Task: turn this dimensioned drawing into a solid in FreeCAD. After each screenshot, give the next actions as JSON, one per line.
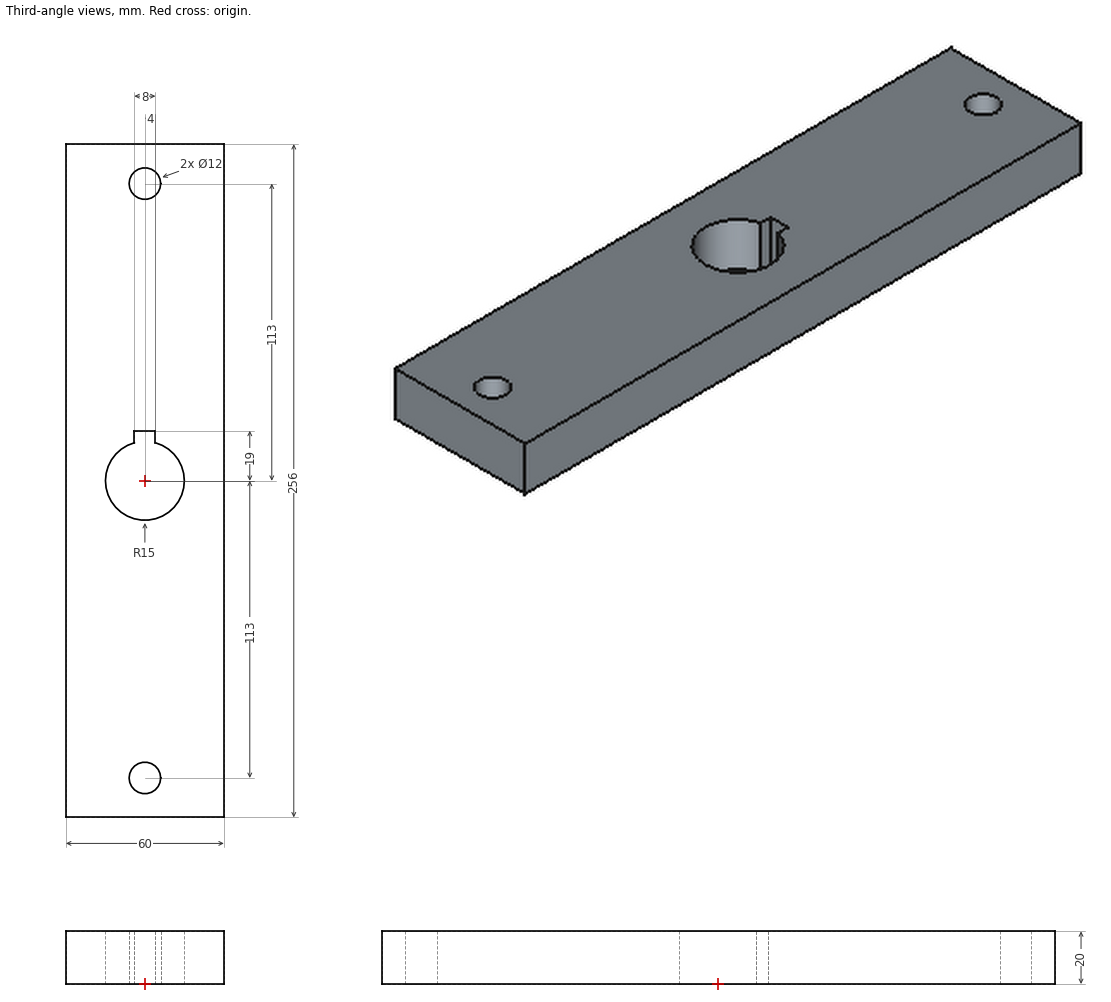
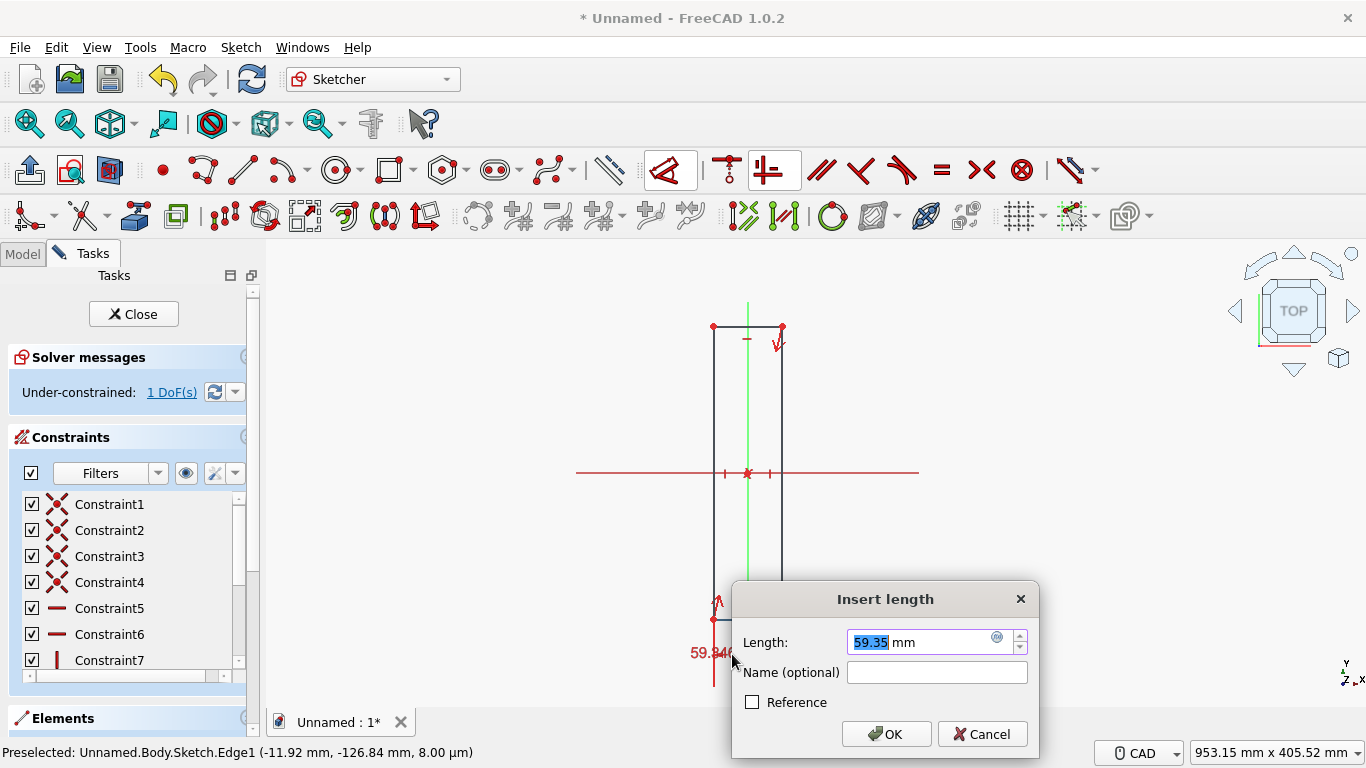
{"action": "type", "text": "60"}
{"action": "key", "text": "Return"}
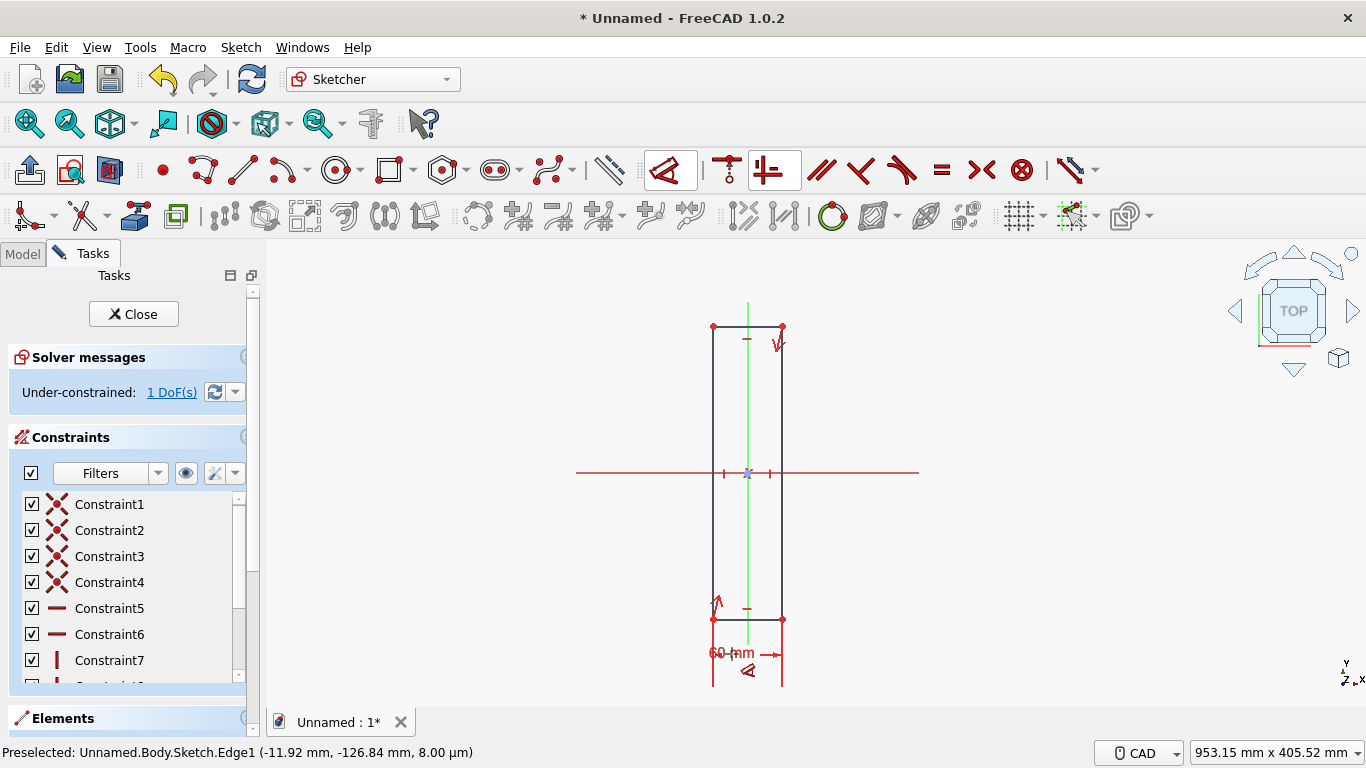
{"action": "left_click", "coordinate": [782, 532]}
{"action": "left_click", "coordinate": [816, 406]}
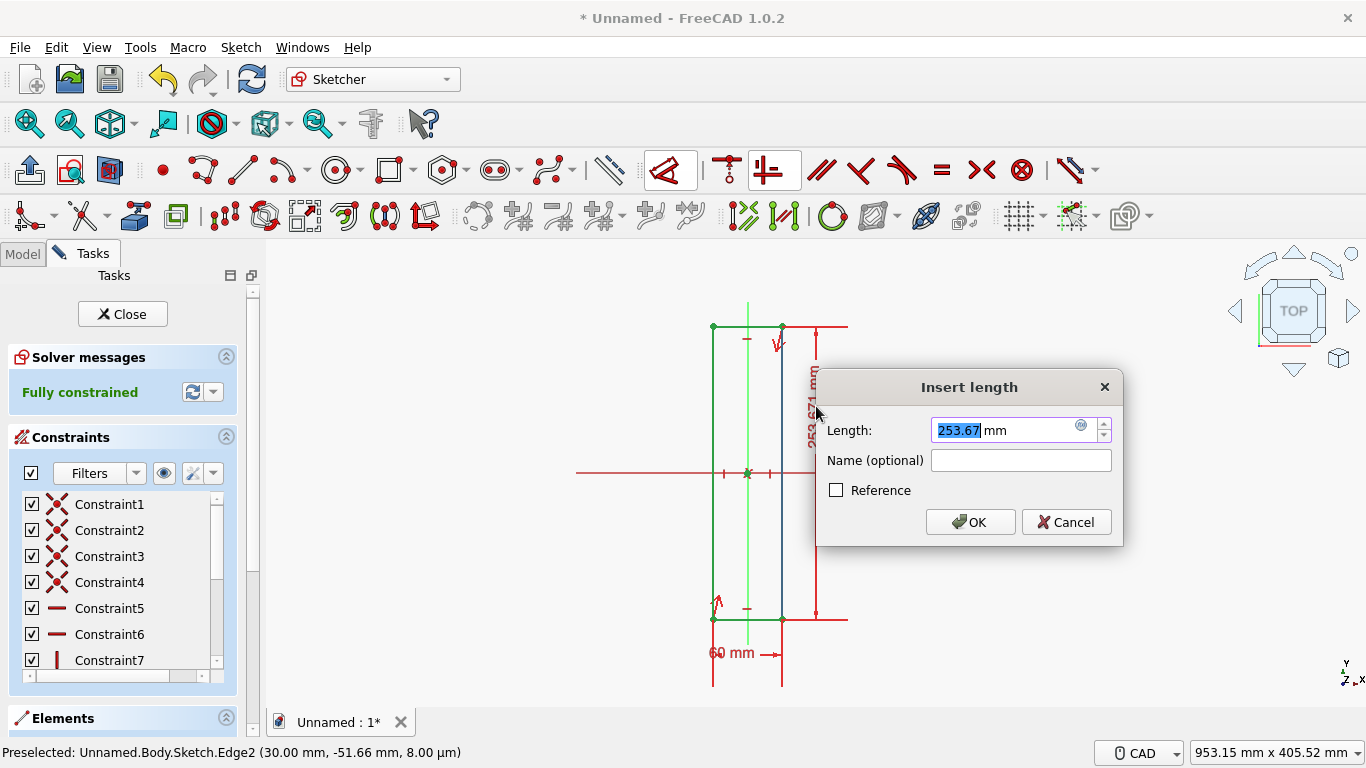
{"action": "type", "text": "256"}
{"action": "key", "text": "Return"}
{"action": "key", "text": "Escape"}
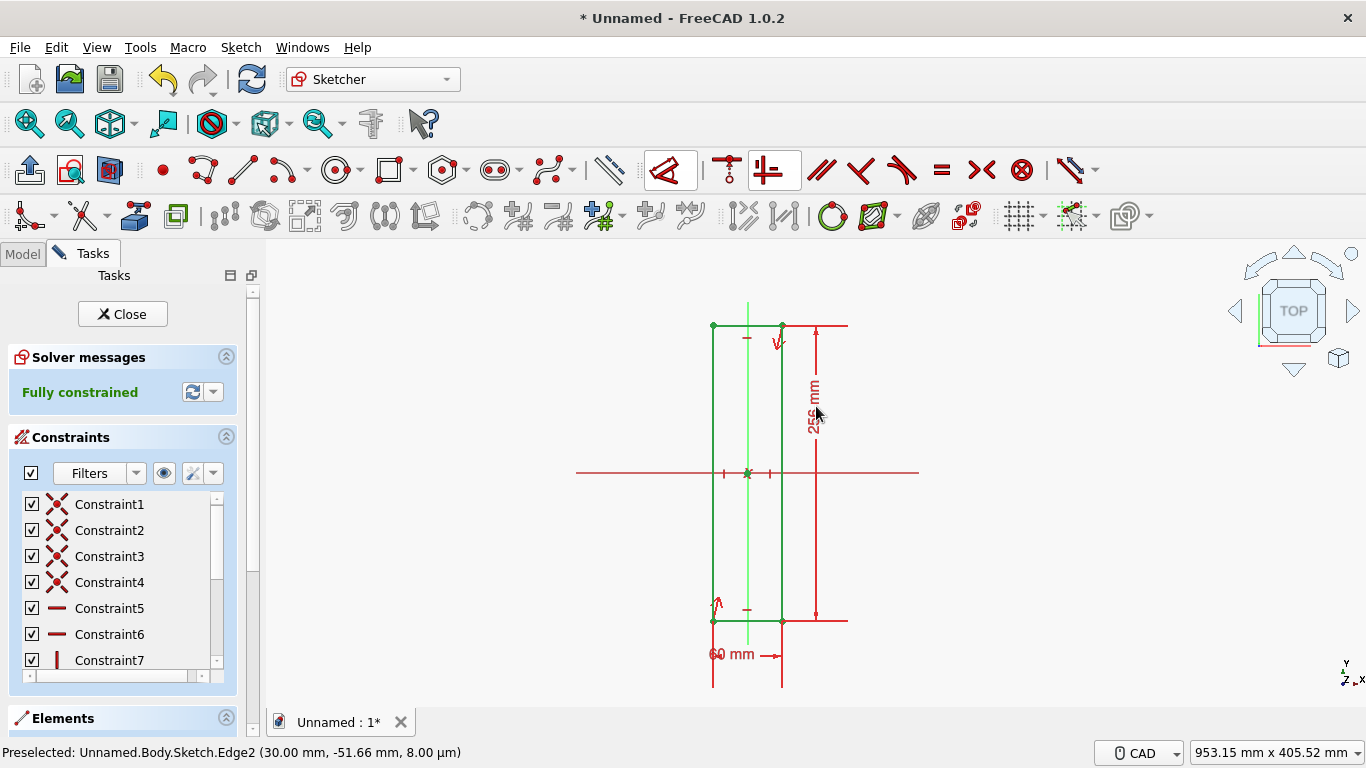
{"action": "left_click", "coordinate": [123, 314]}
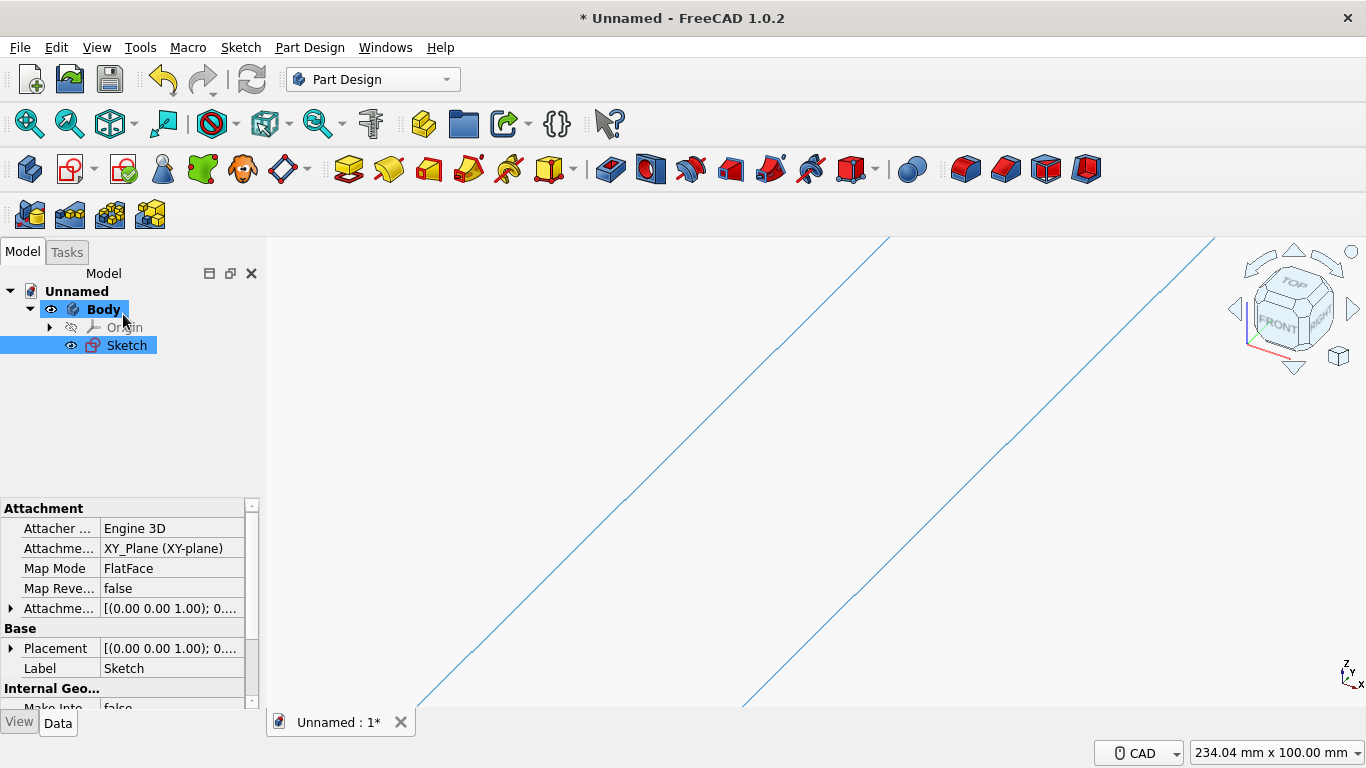
{"action": "left_click", "coordinate": [350, 170]}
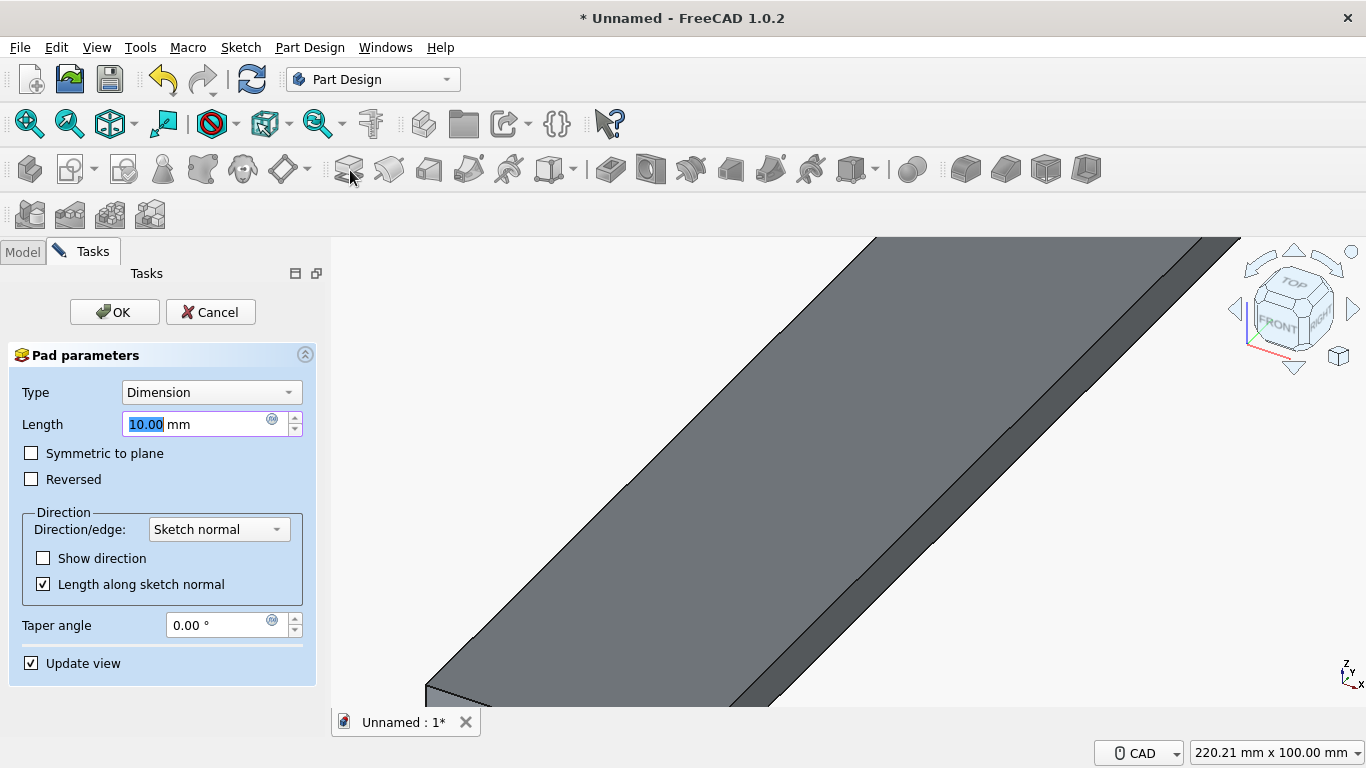
{"action": "type", "text": "20"}
{"action": "key", "text": "Tab"}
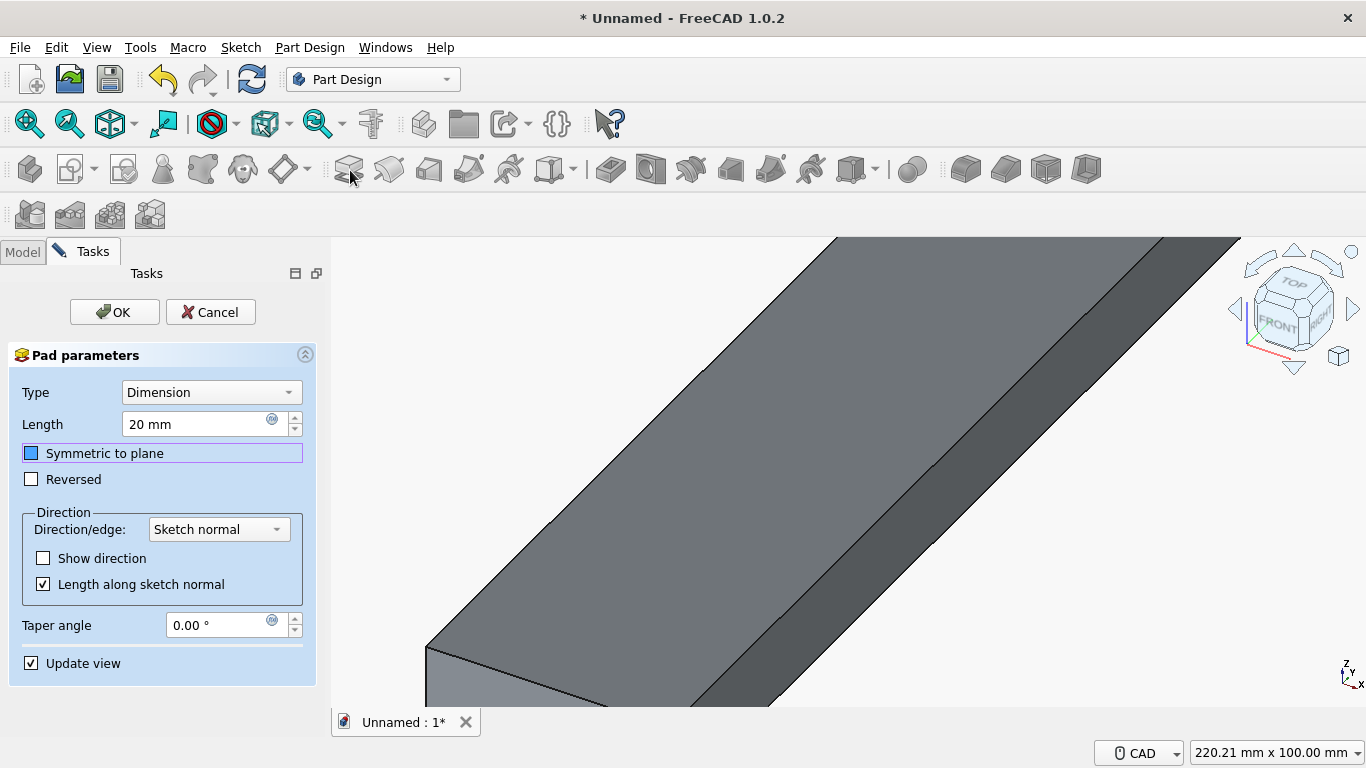
{"action": "left_click", "coordinate": [115, 312]}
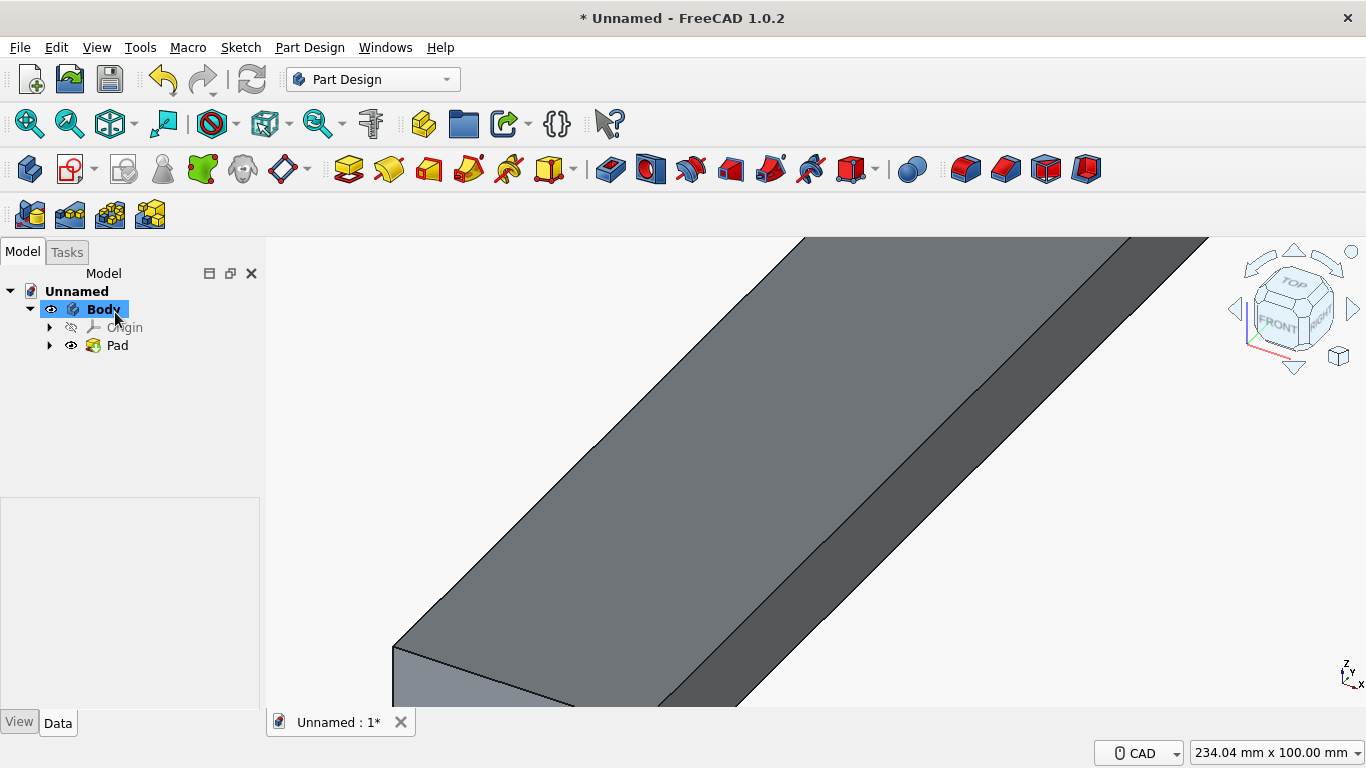
{"action": "left_click", "coordinate": [30, 124]}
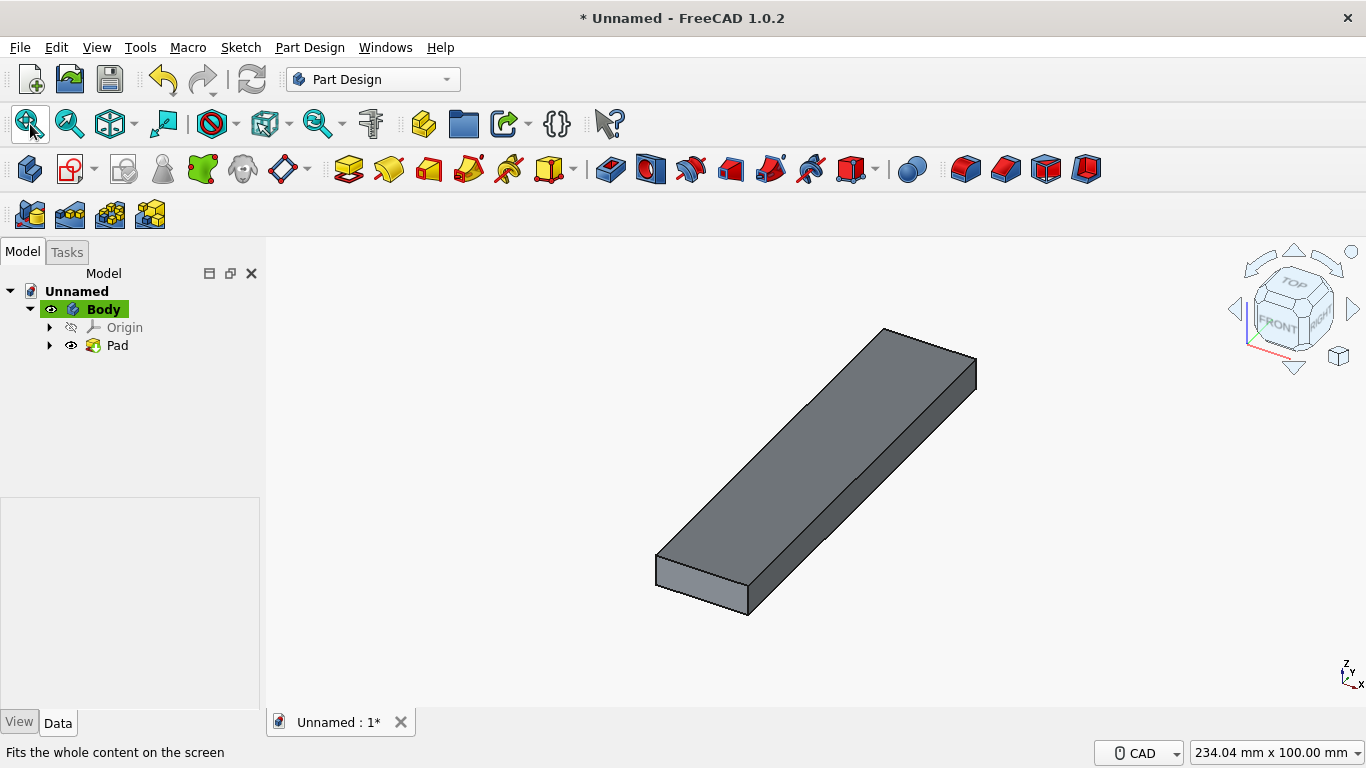
{"action": "left_click", "coordinate": [881, 392]}